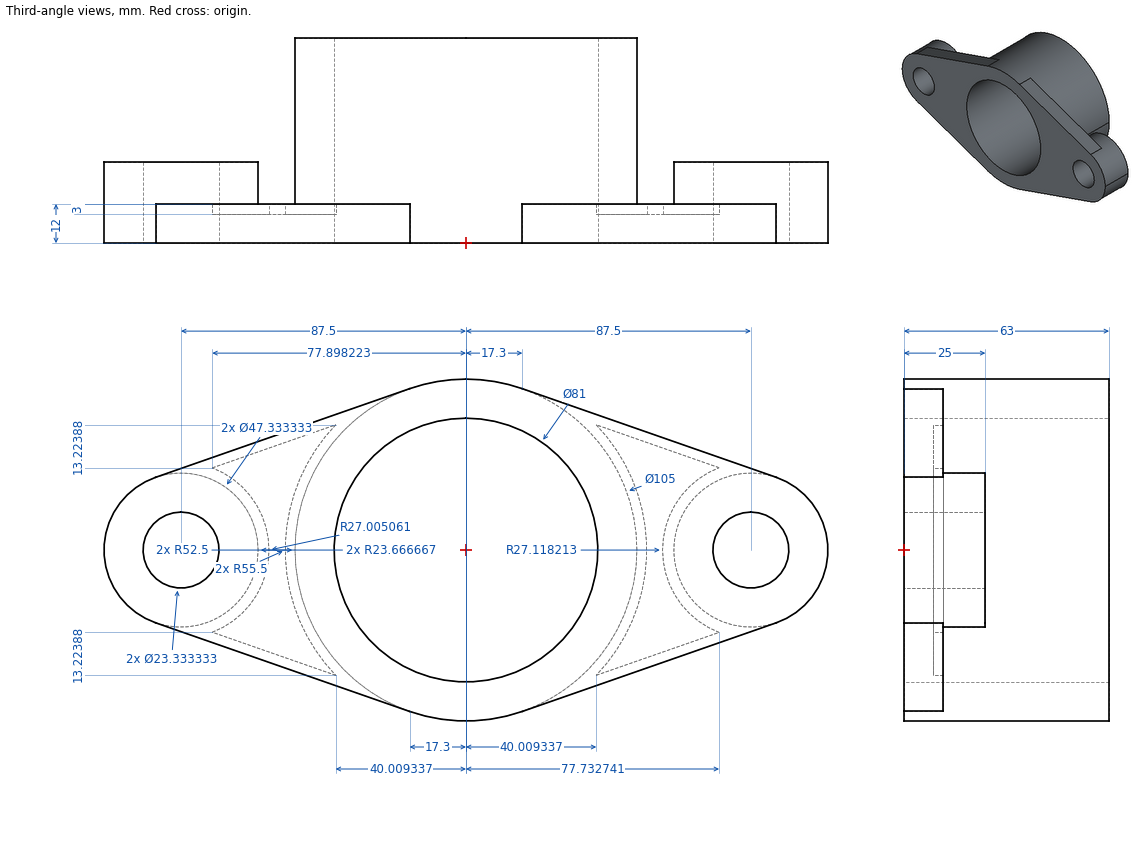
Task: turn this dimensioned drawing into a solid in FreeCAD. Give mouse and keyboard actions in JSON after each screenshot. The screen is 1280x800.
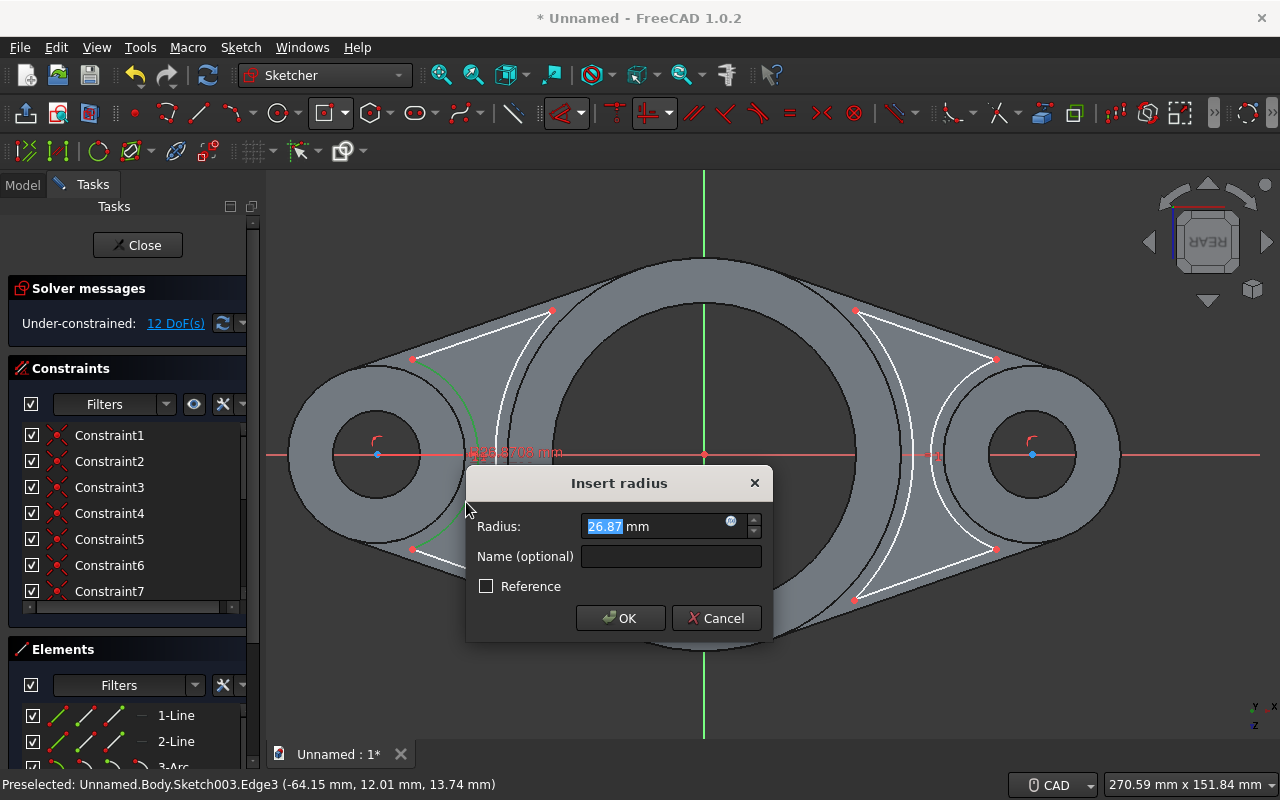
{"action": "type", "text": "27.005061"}
{"action": "key", "text": "Return"}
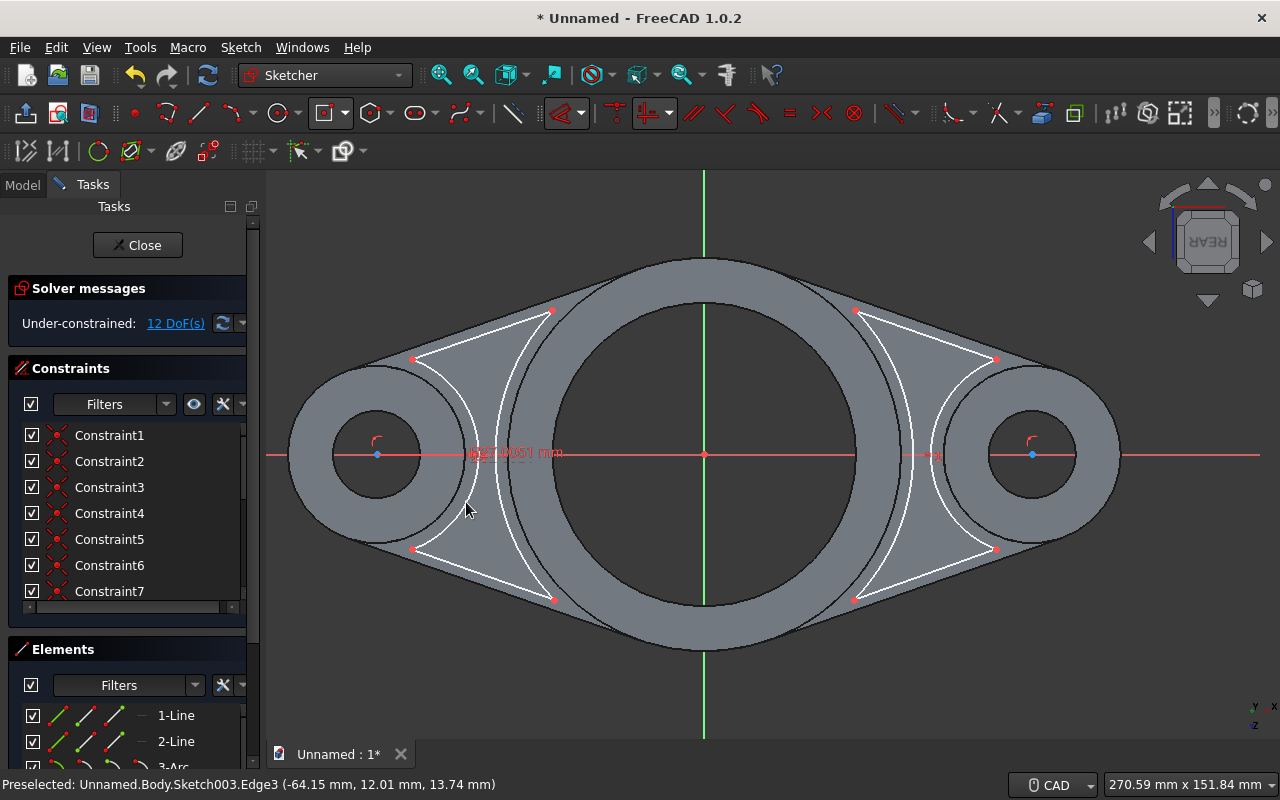
{"action": "left_click", "coordinate": [505, 393]}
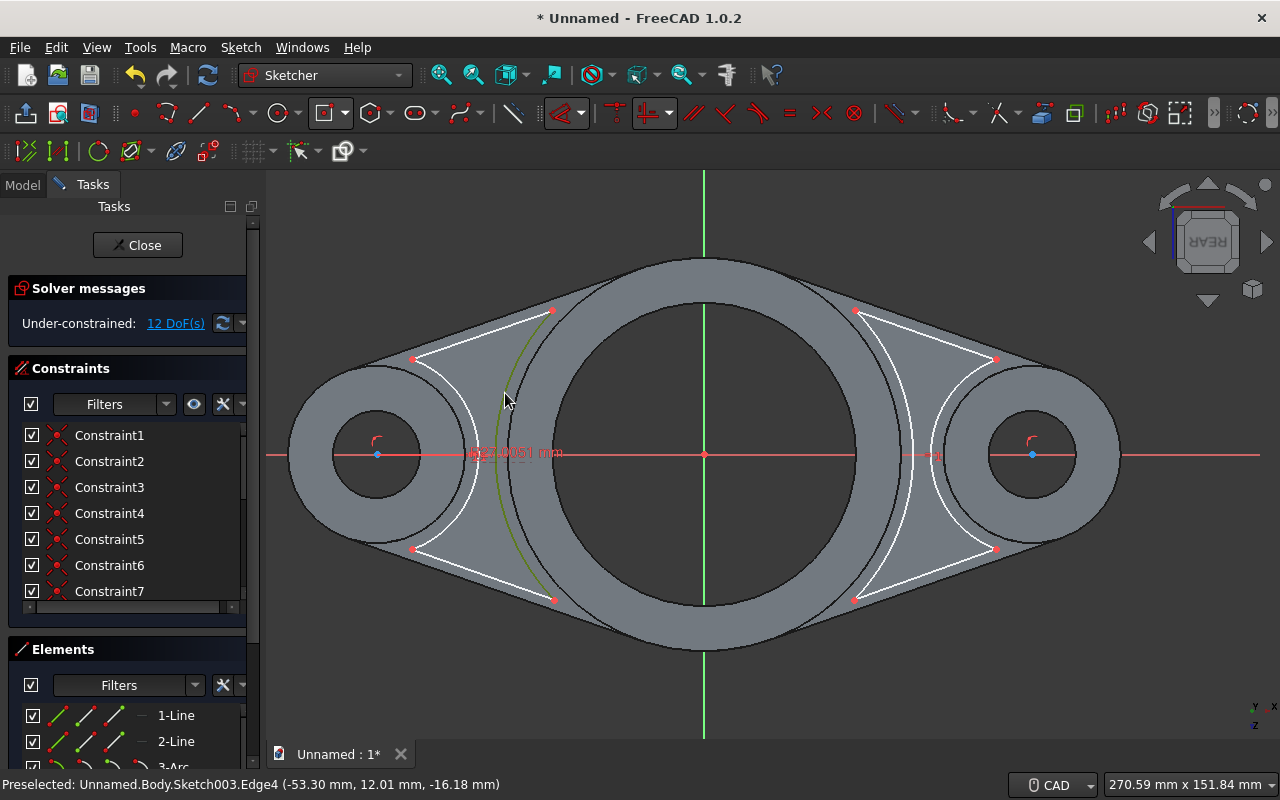
{"action": "key", "text": "k r"}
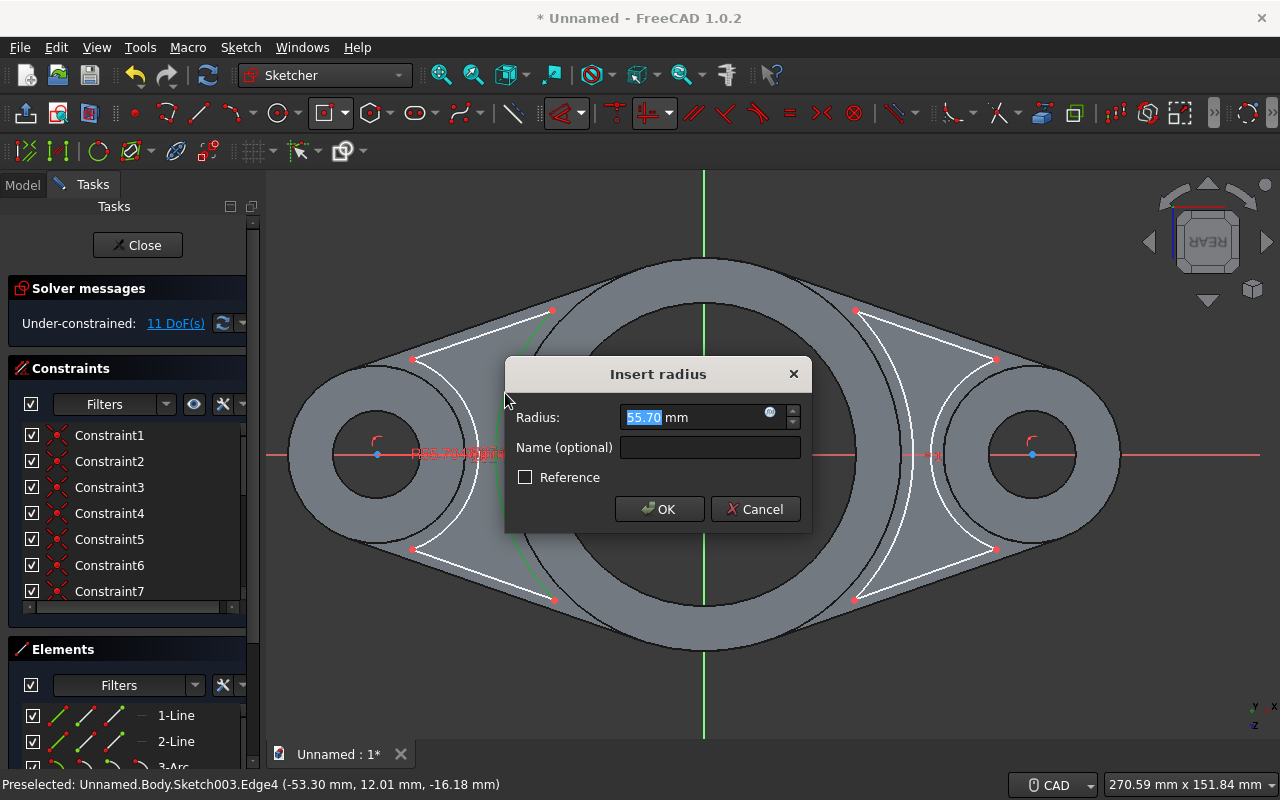
{"action": "type", "text": "55.5"}
{"action": "key", "text": "Return"}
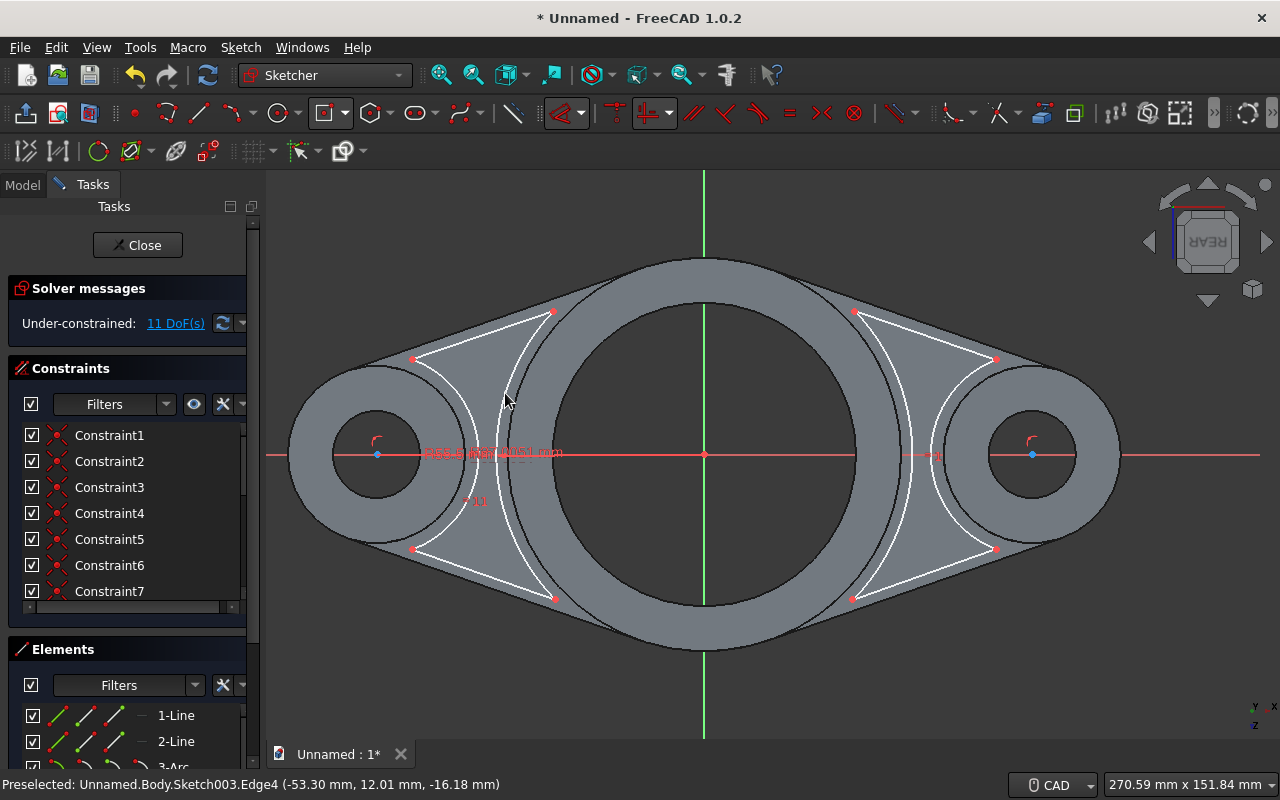
{"action": "left_click", "coordinate": [942, 408]}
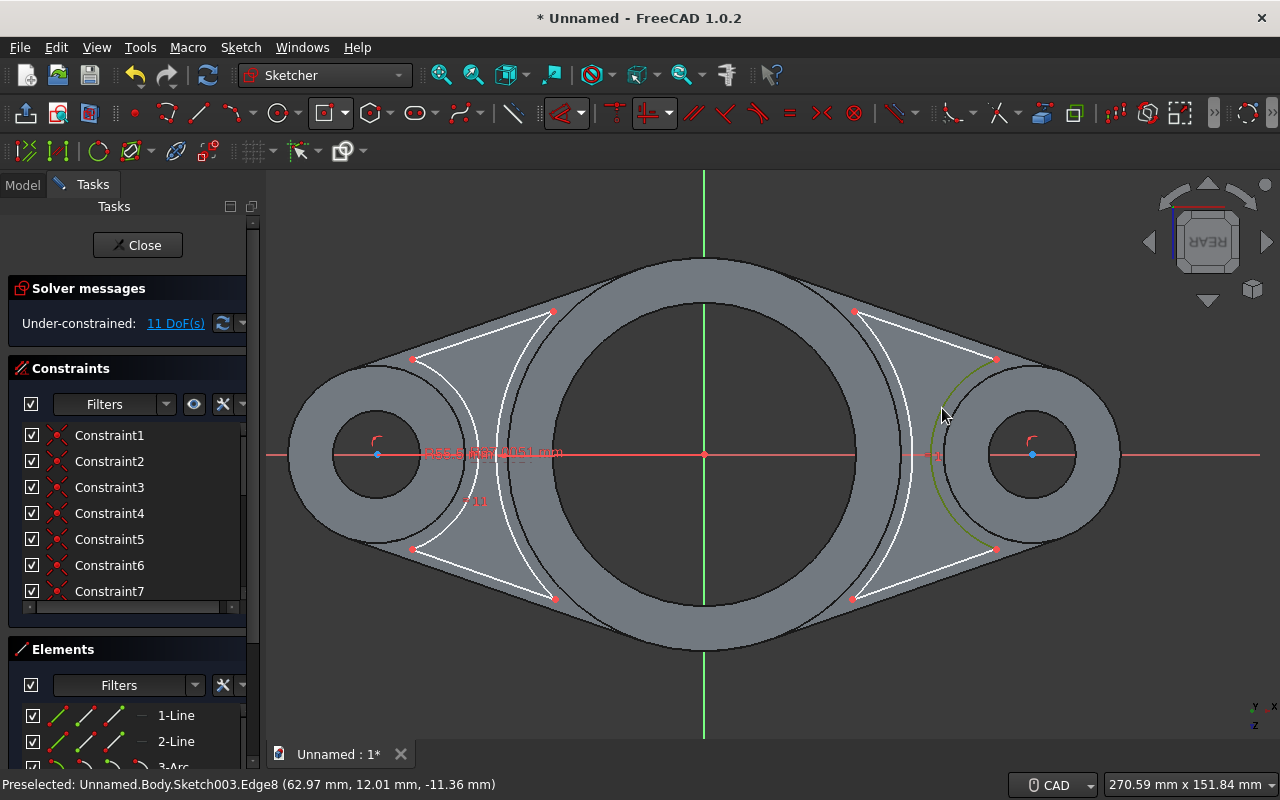
{"action": "left_click", "coordinate": [584, 114]}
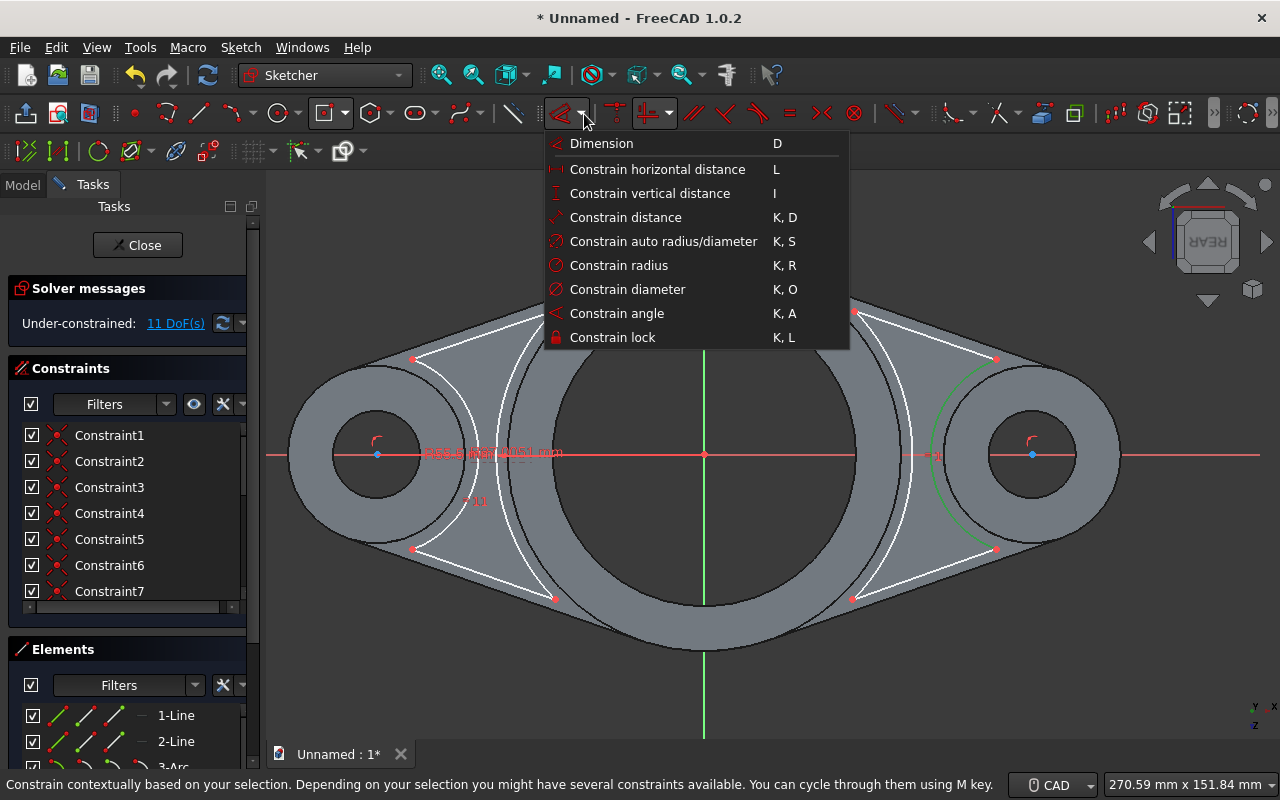
{"action": "left_click", "coordinate": [697, 265]}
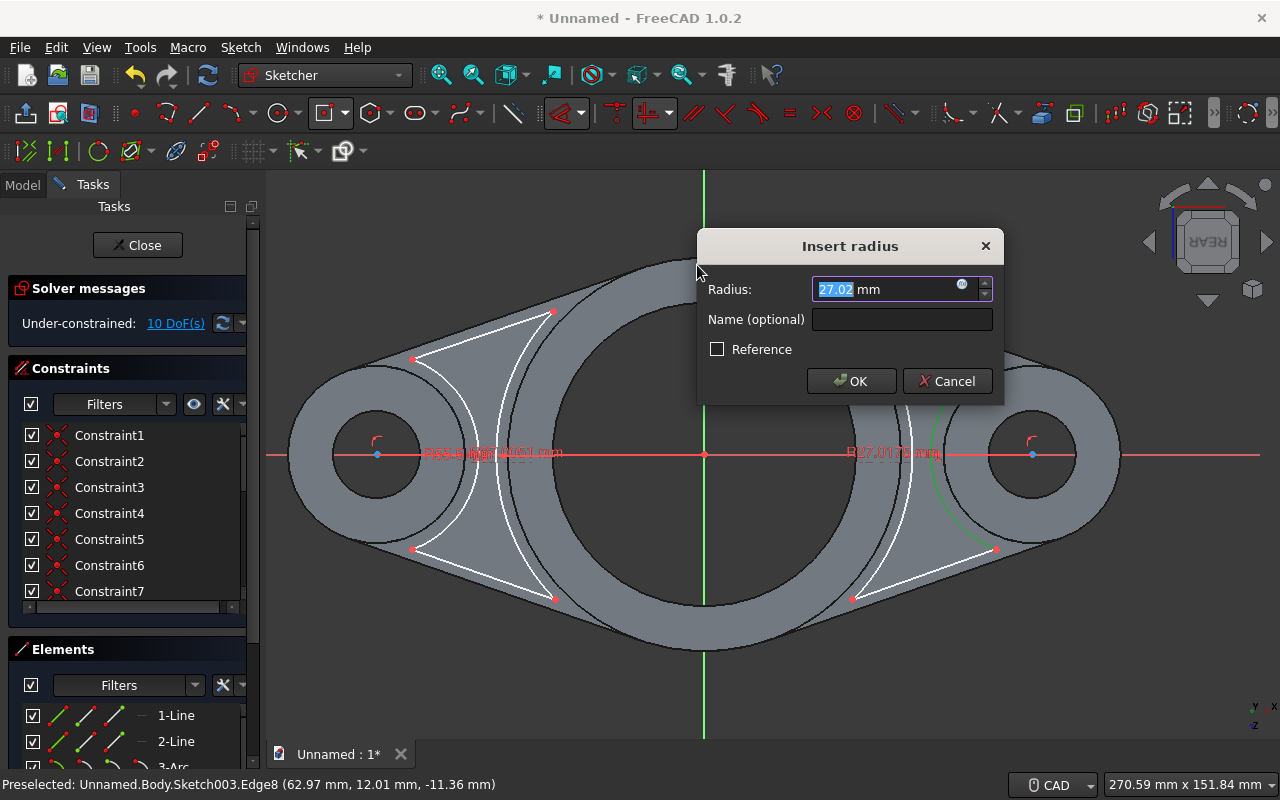
{"action": "type", "text": "27.118213"}
{"action": "key", "text": "Return"}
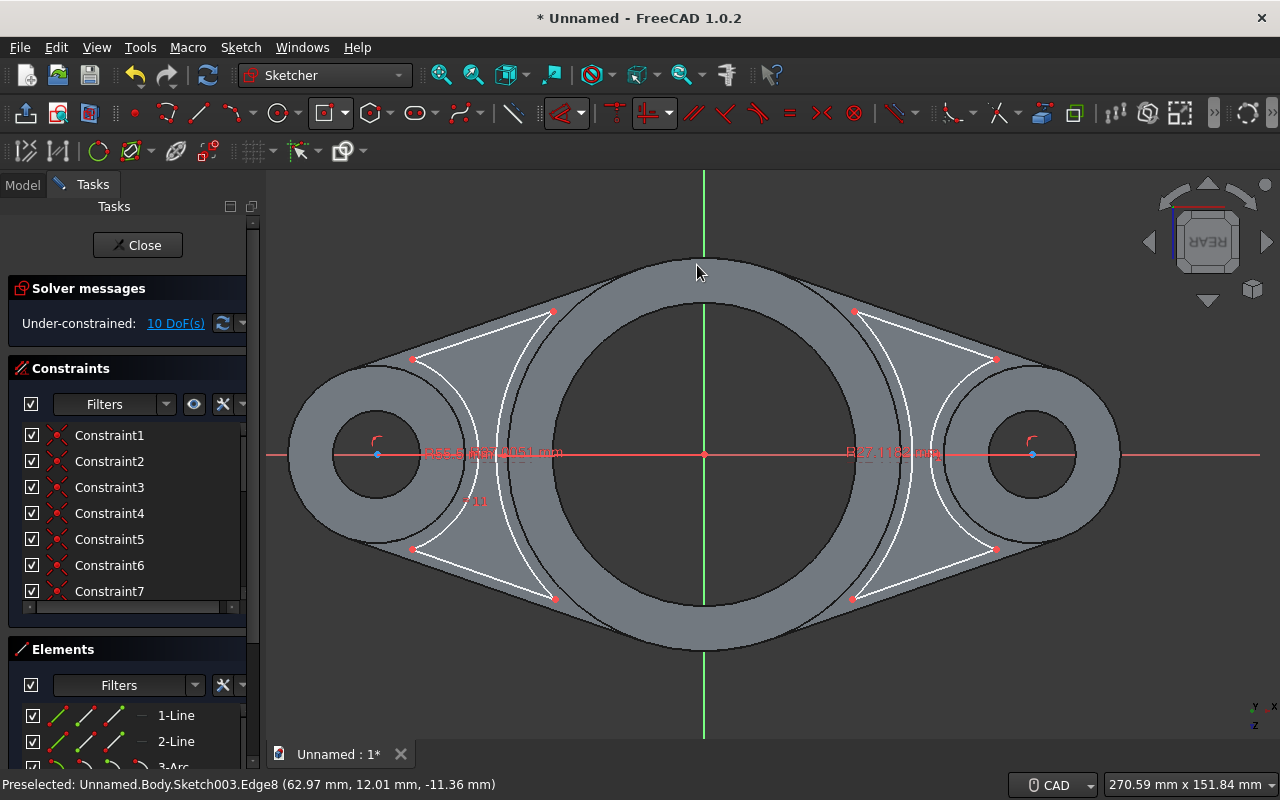
{"action": "left_click", "coordinate": [377, 454]}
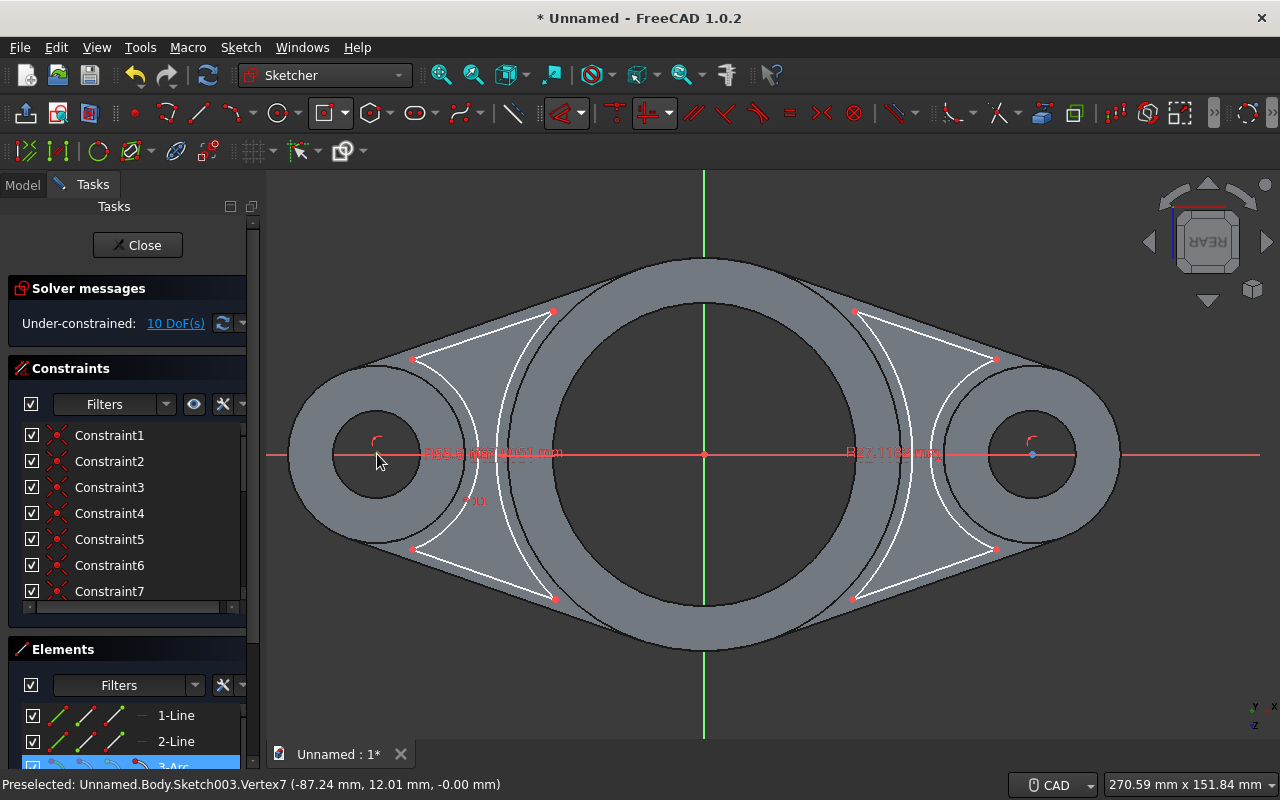
{"action": "key", "text": "l"}